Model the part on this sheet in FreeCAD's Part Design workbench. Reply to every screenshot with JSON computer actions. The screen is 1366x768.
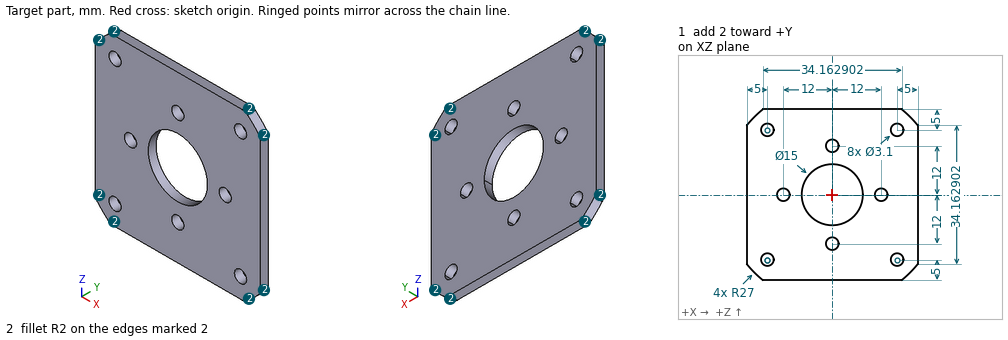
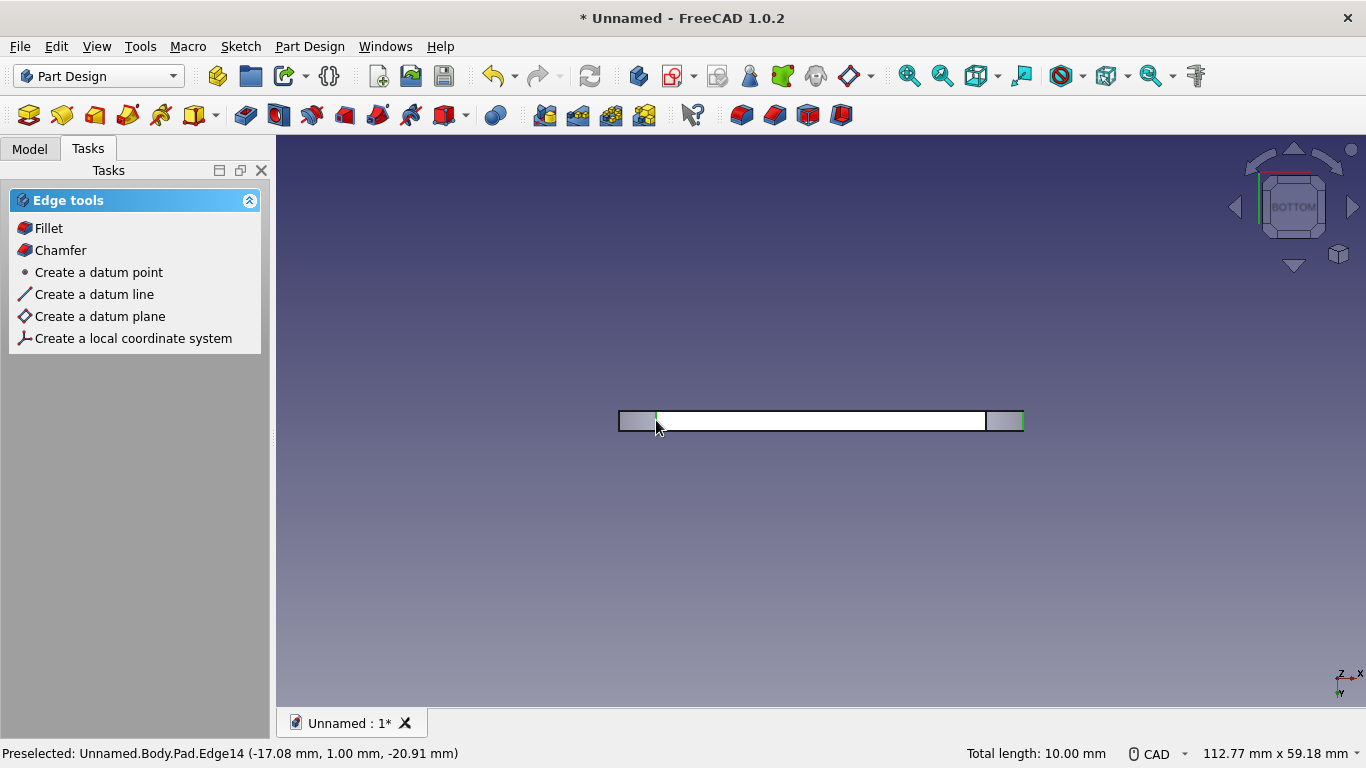
{"action": "left_click", "coordinate": [986, 420], "text": "ctrl"}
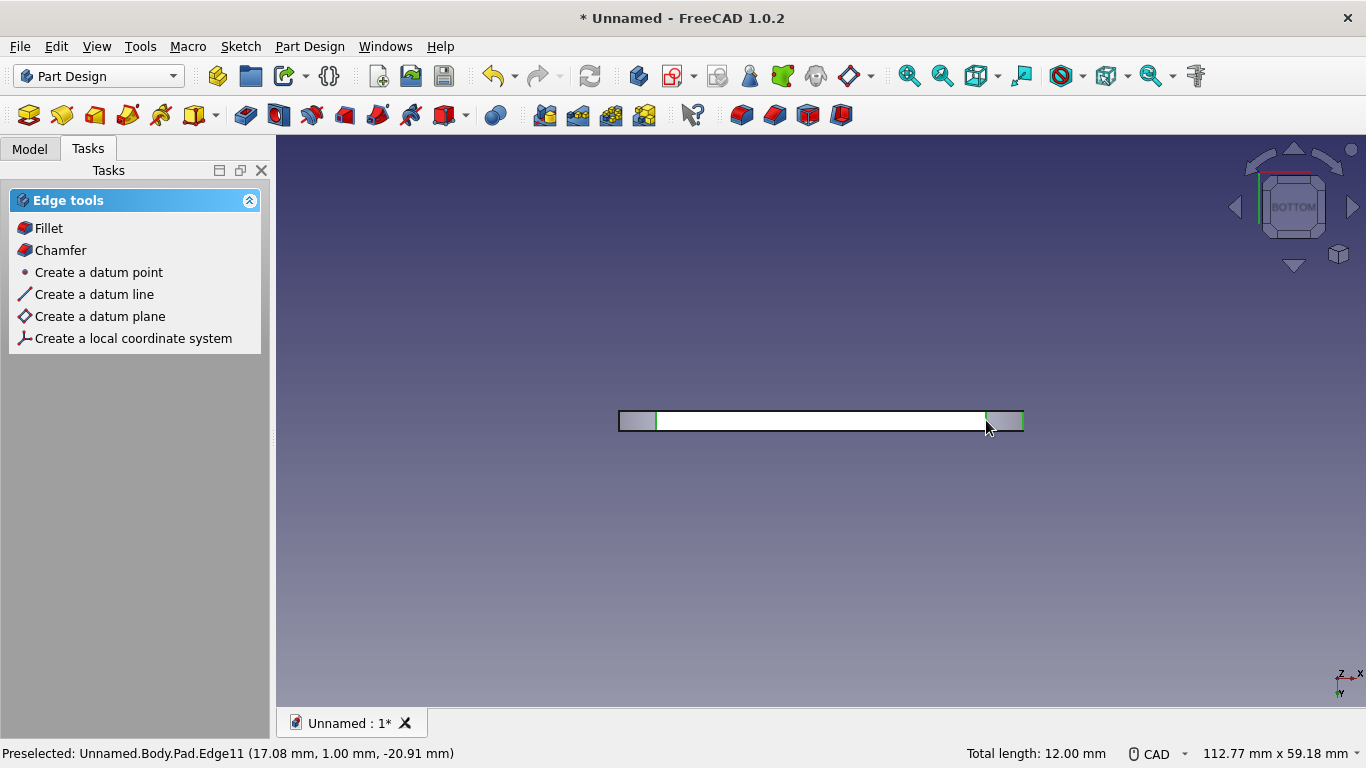
{"action": "scroll", "coordinate": [619, 420], "scroll_direction": "up", "scroll_amount": 4}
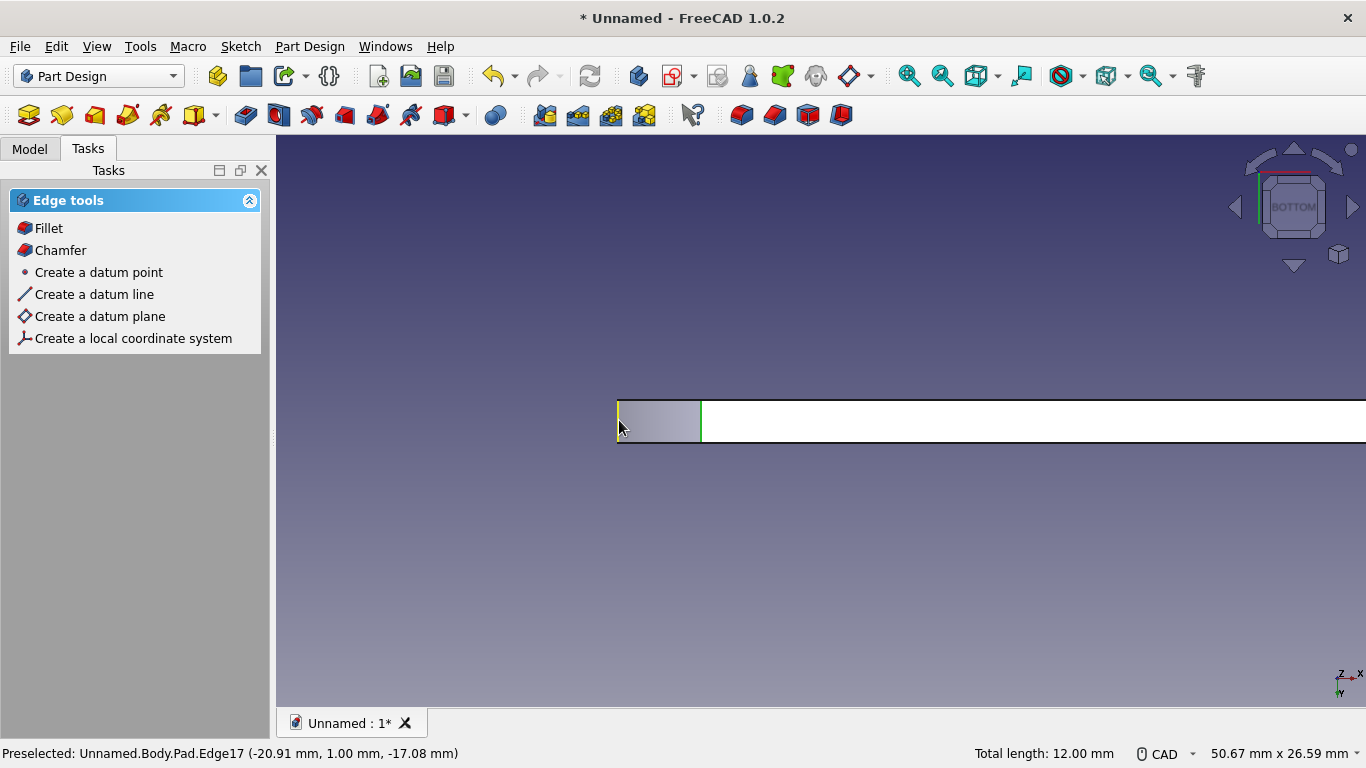
{"action": "left_click", "coordinate": [910, 76]}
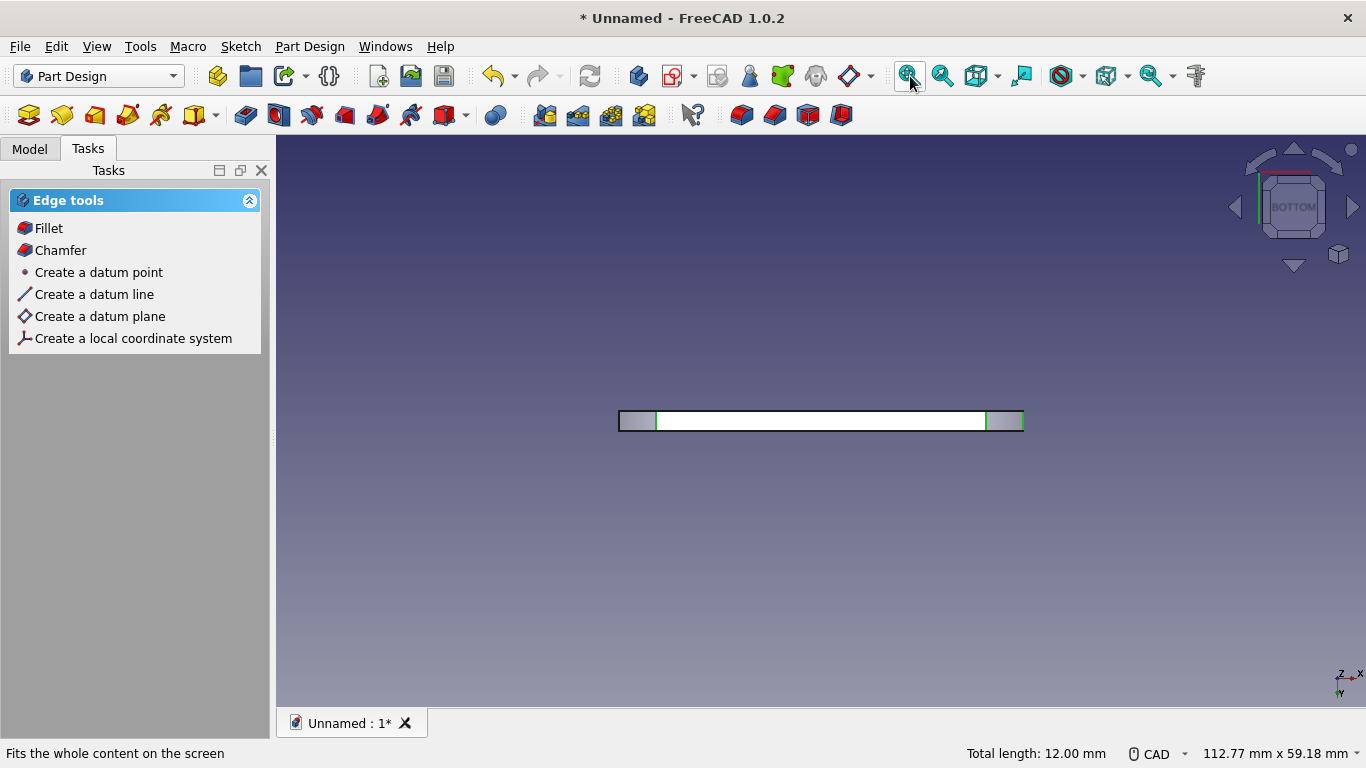
{"action": "key", "text": "4"}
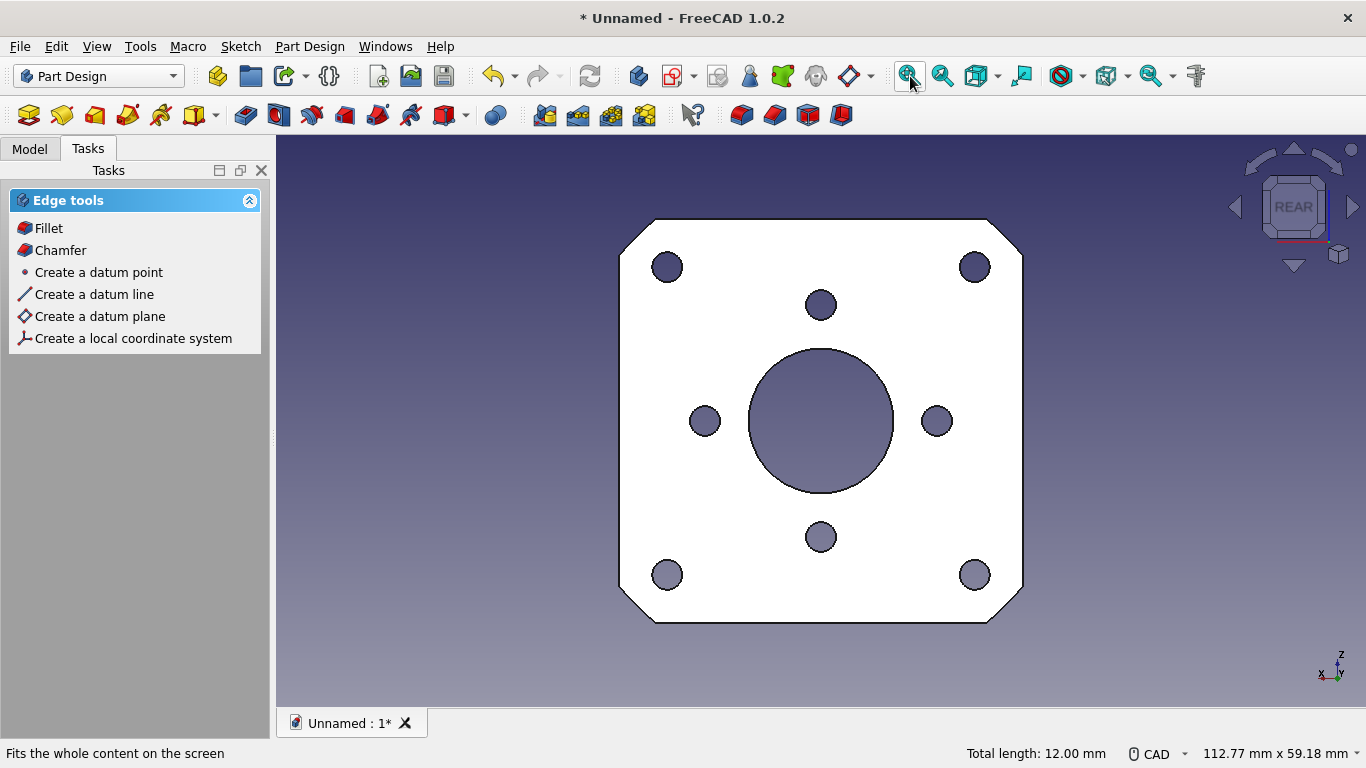
{"action": "scroll", "coordinate": [1023, 255], "scroll_direction": "up", "scroll_amount": 4}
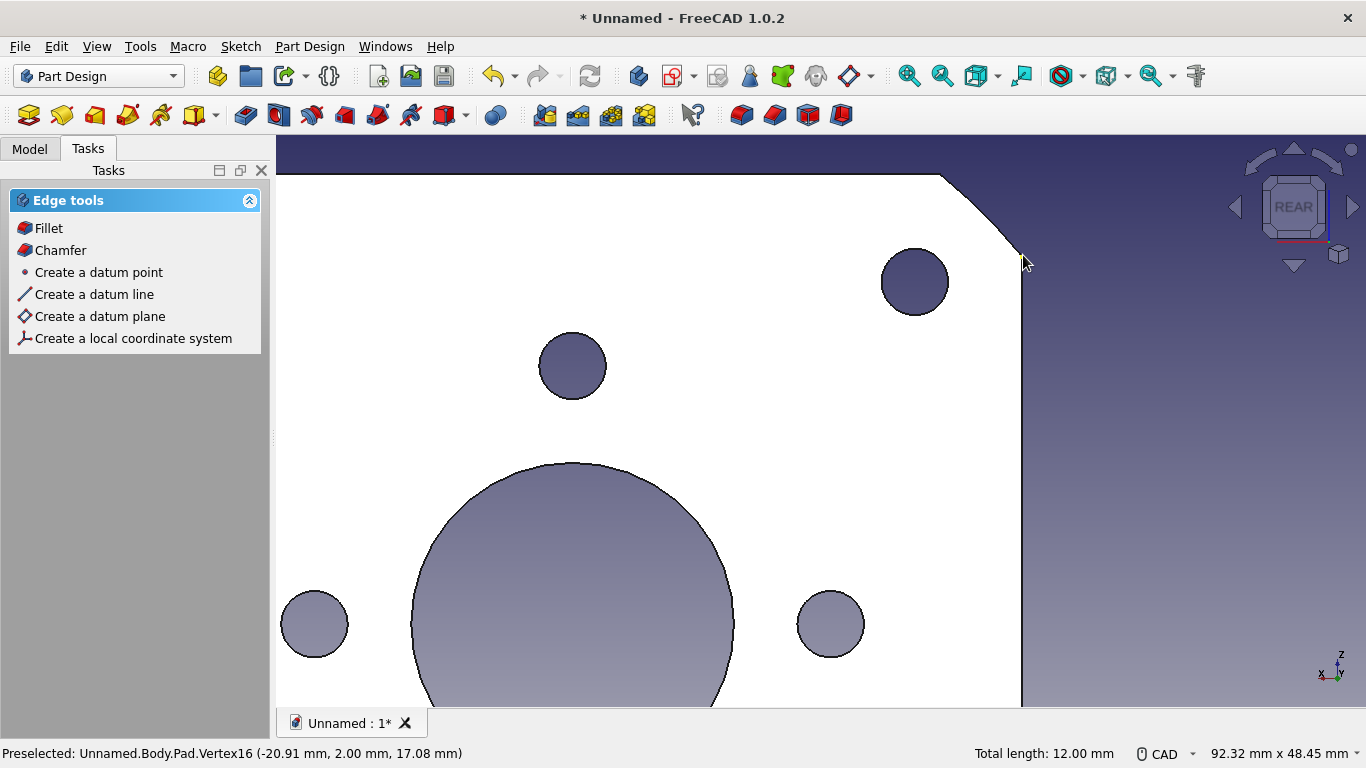
{"action": "left_click", "coordinate": [910, 76]}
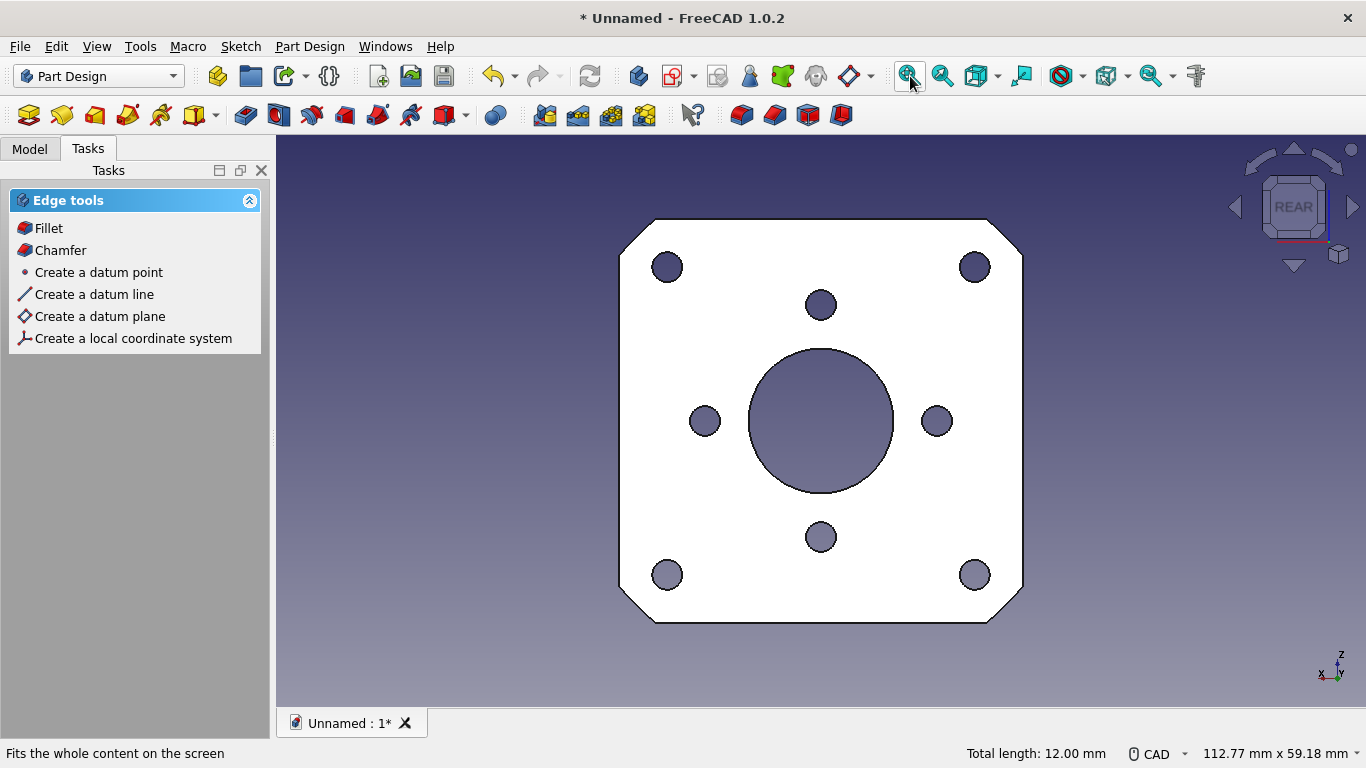
{"action": "key", "text": "6"}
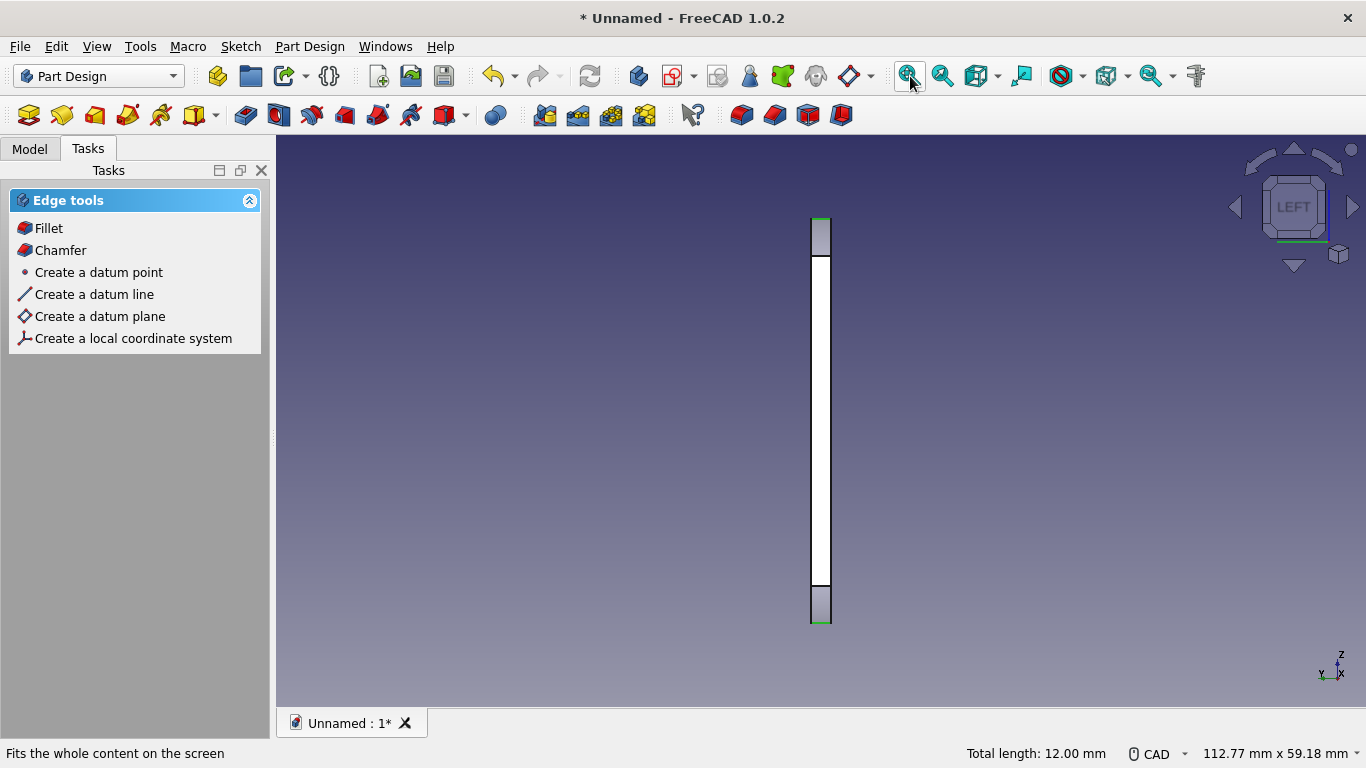
{"action": "left_click", "coordinate": [821, 255], "text": "ctrl"}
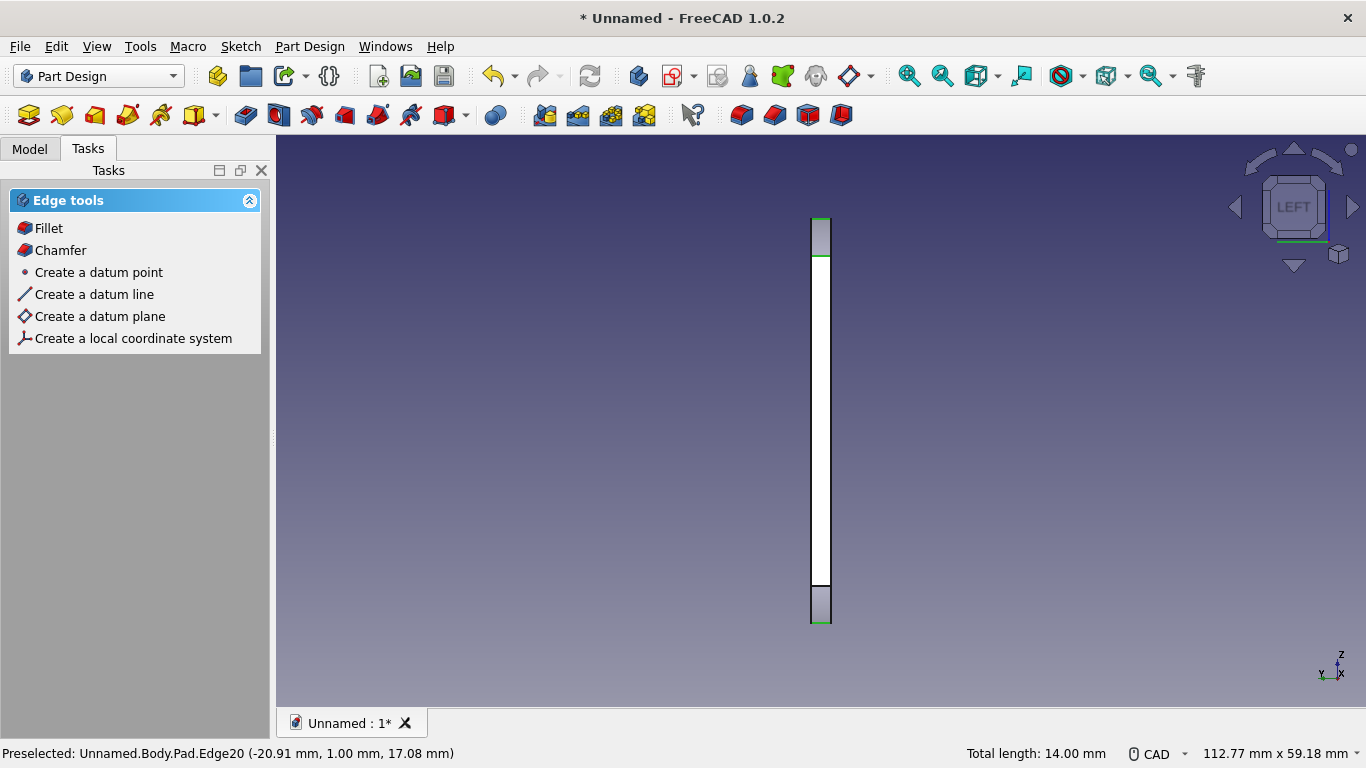
{"action": "left_click", "coordinate": [821, 585], "text": "ctrl"}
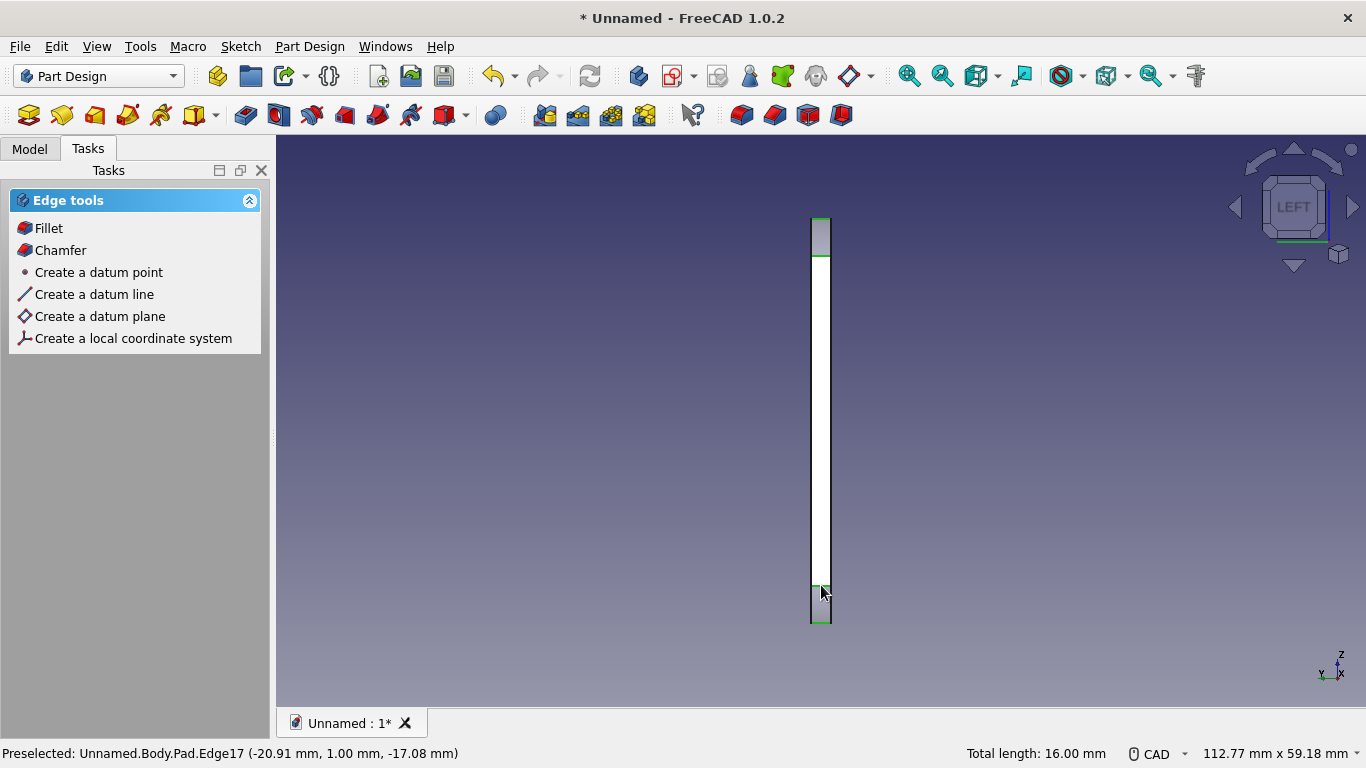
{"action": "left_click", "coordinate": [742, 116]}